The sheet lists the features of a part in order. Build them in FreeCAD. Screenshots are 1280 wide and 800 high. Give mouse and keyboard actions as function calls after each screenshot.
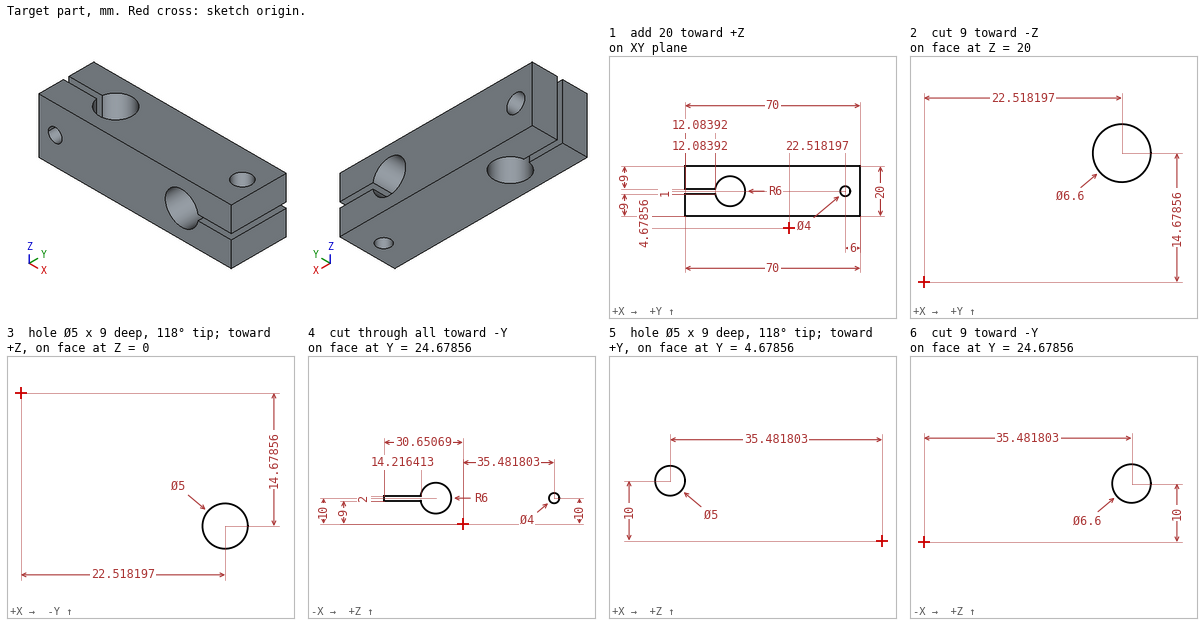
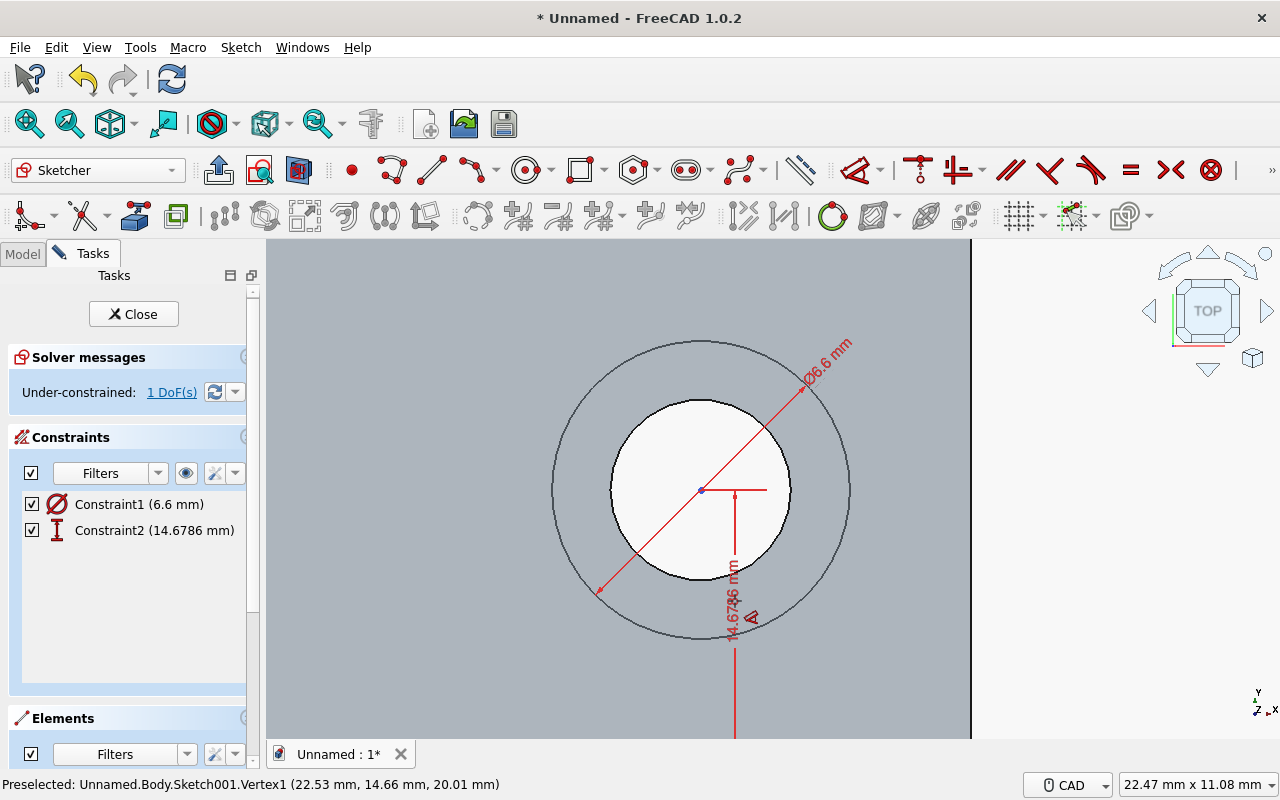
click(701, 490)
click(497, 456)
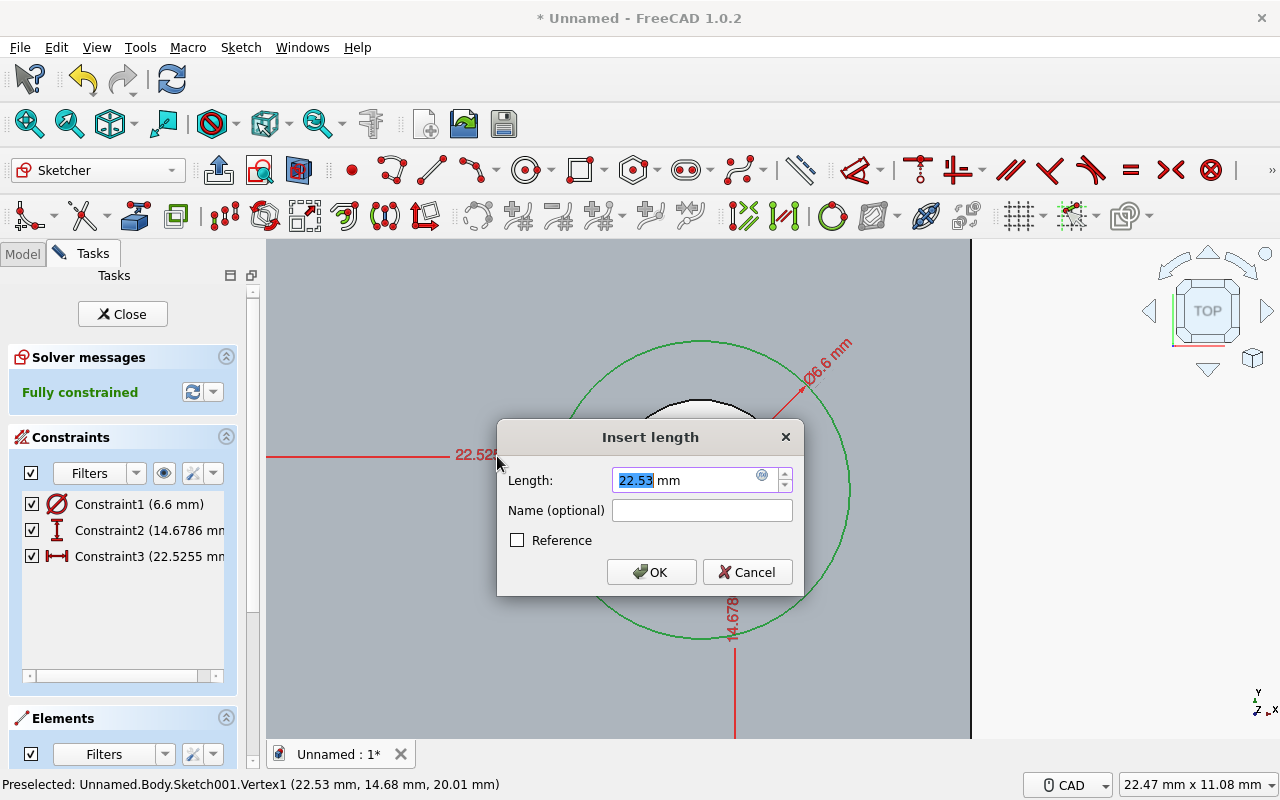
text(22.518197)
key(Return)
key(Escape)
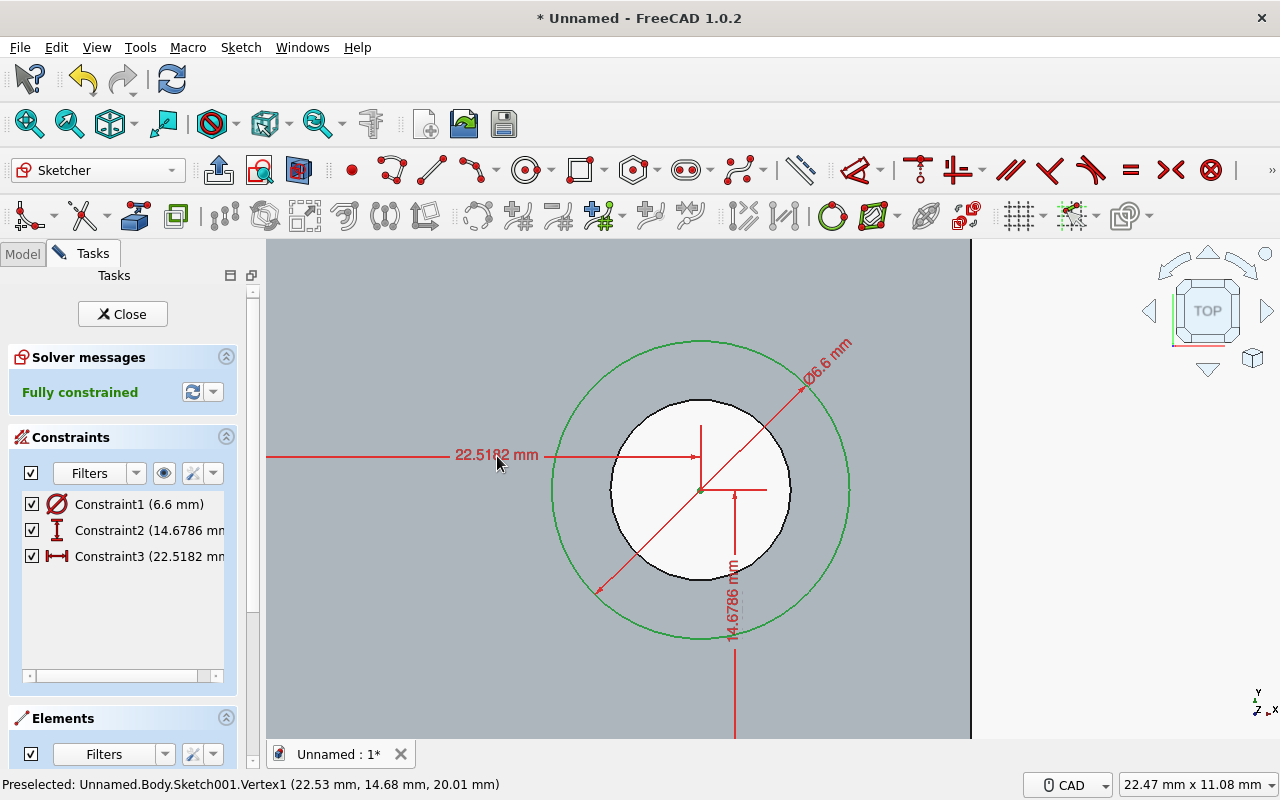
click(123, 314)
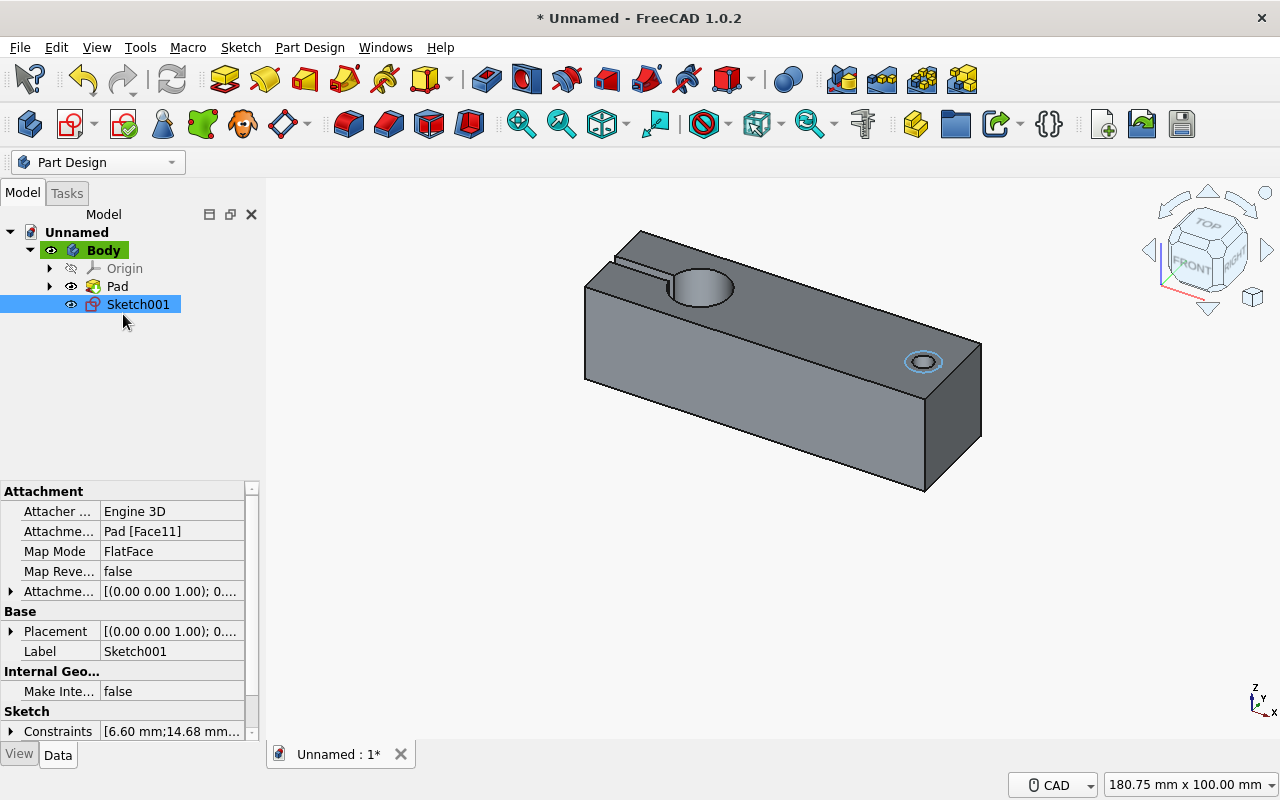
click(488, 80)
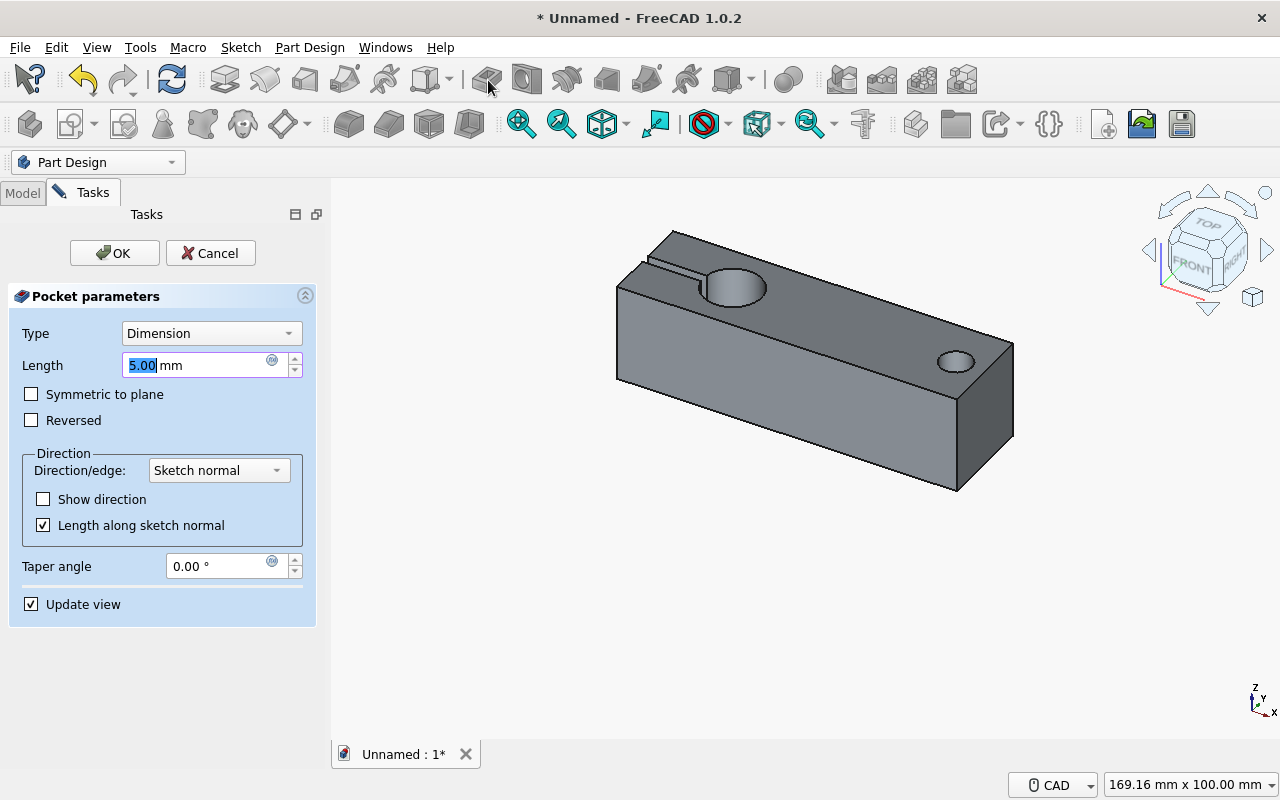
text(9)
key(Tab)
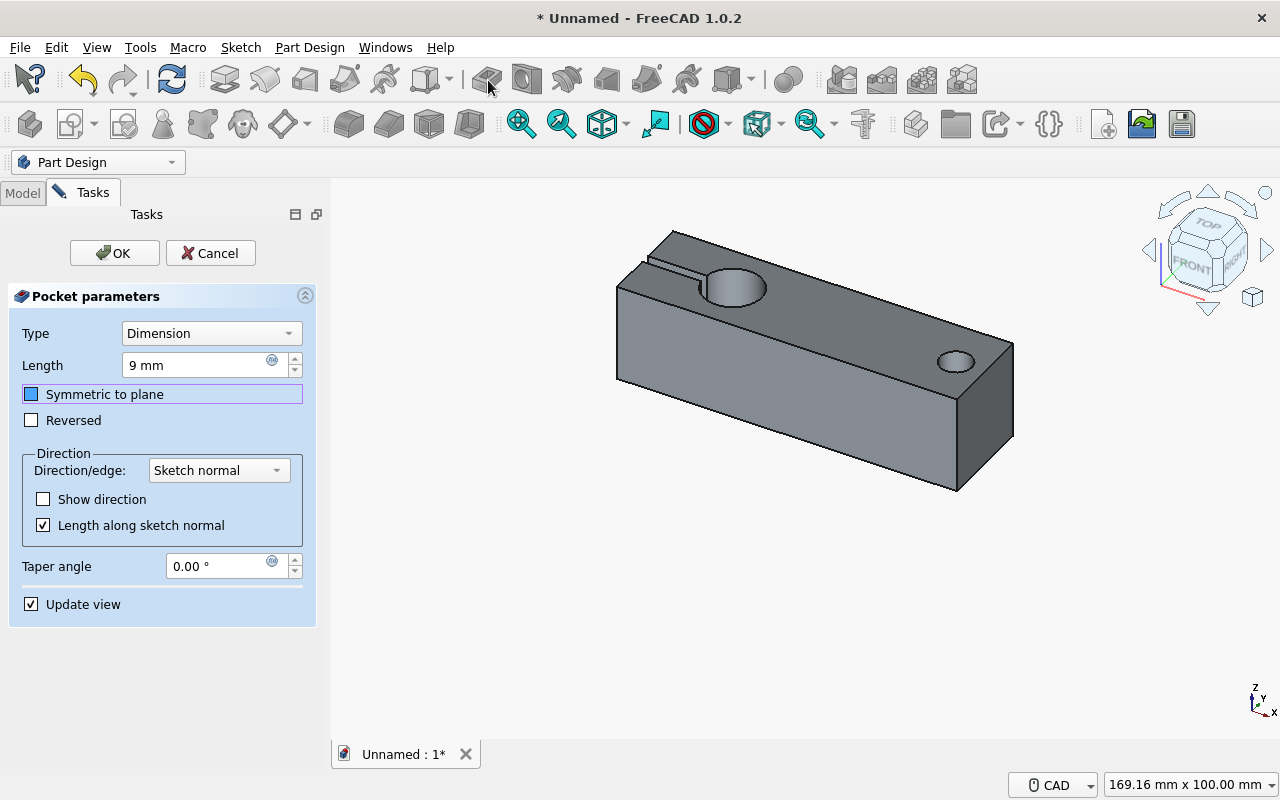
click(115, 253)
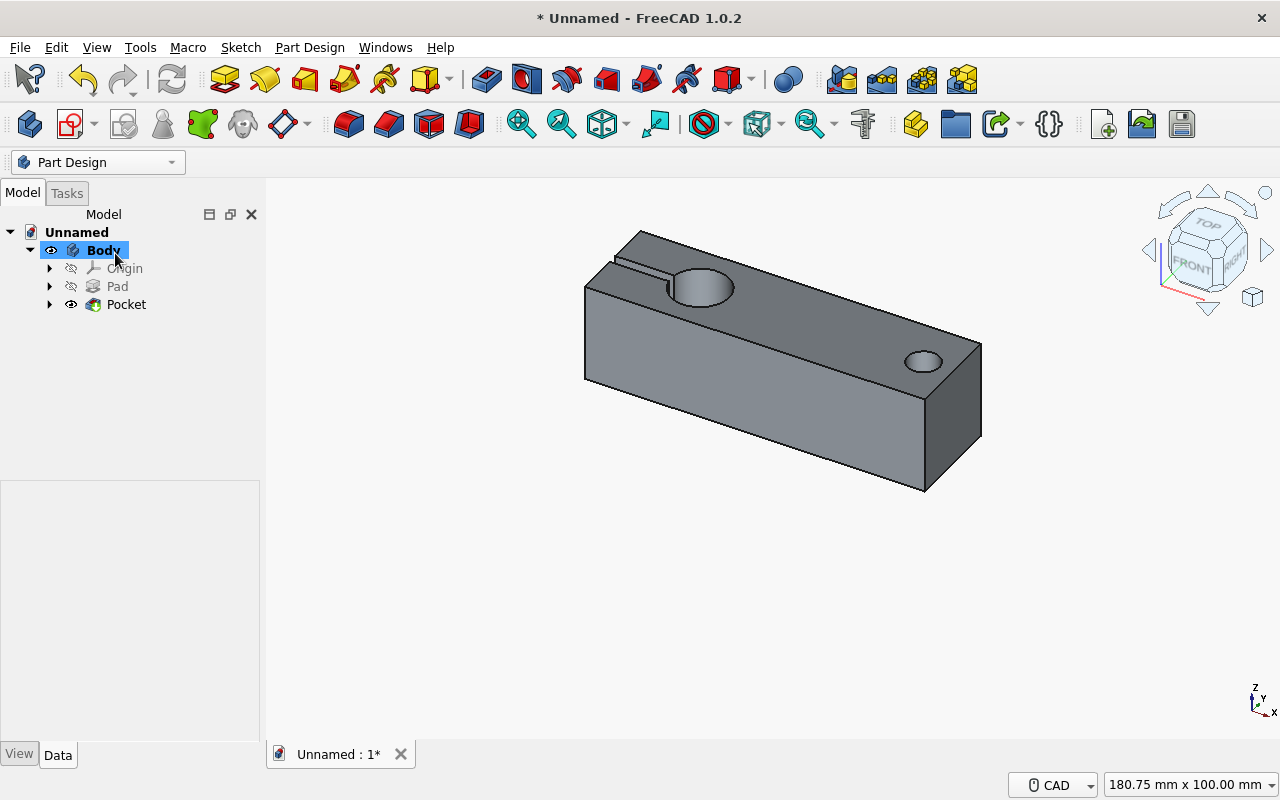
key(5)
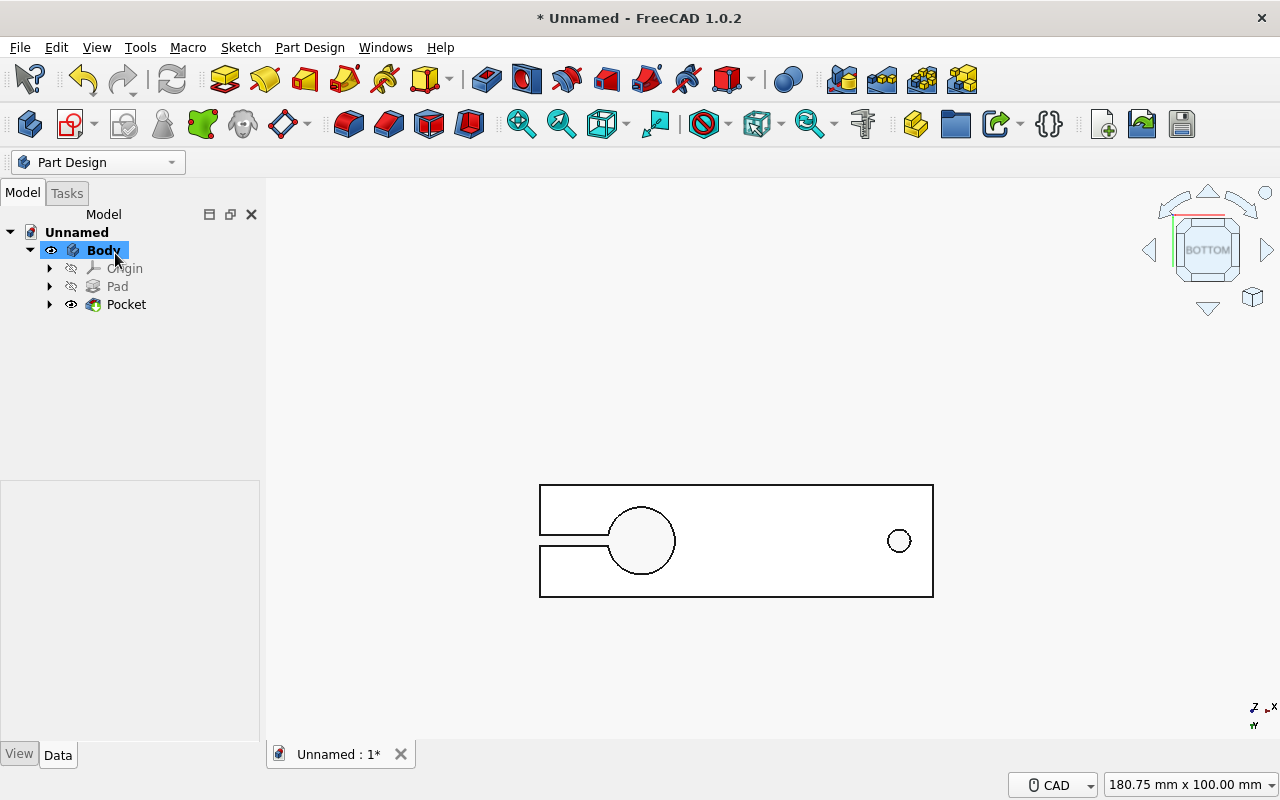
click(522, 124)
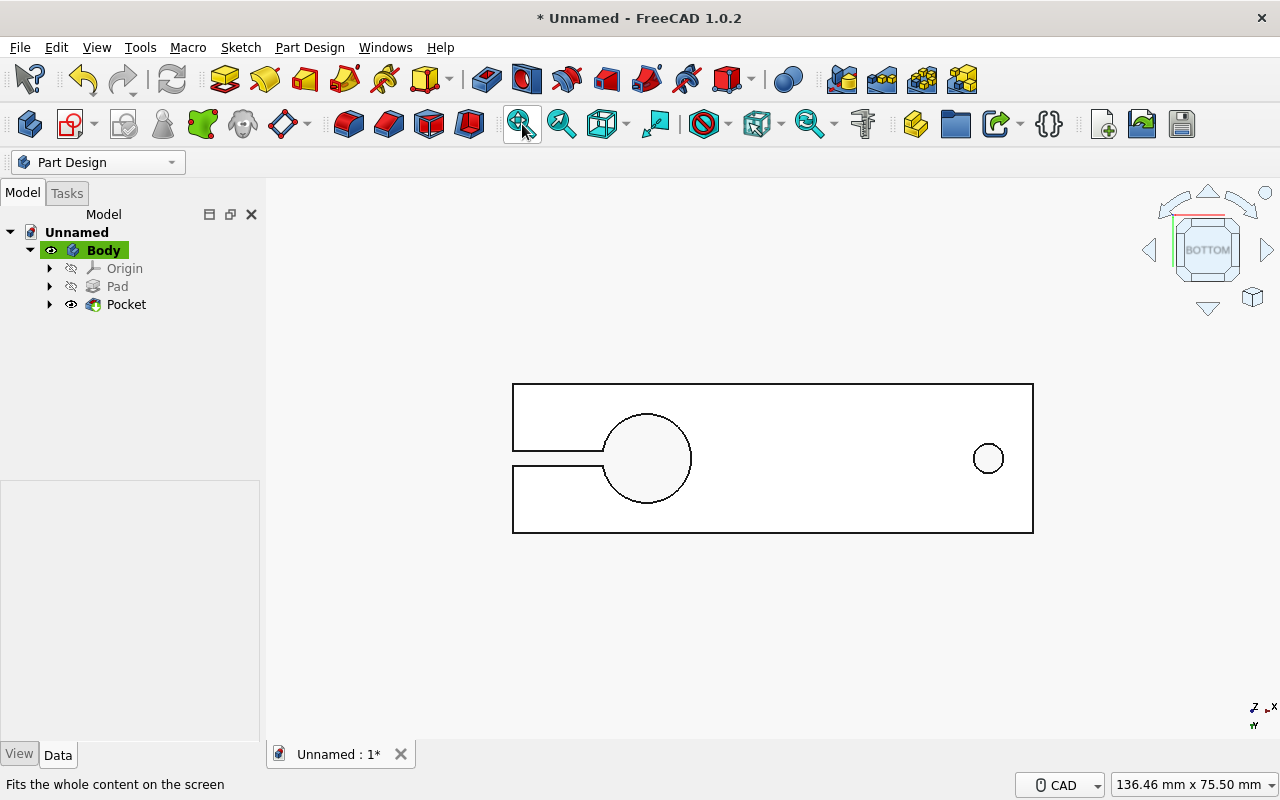
click(847, 457)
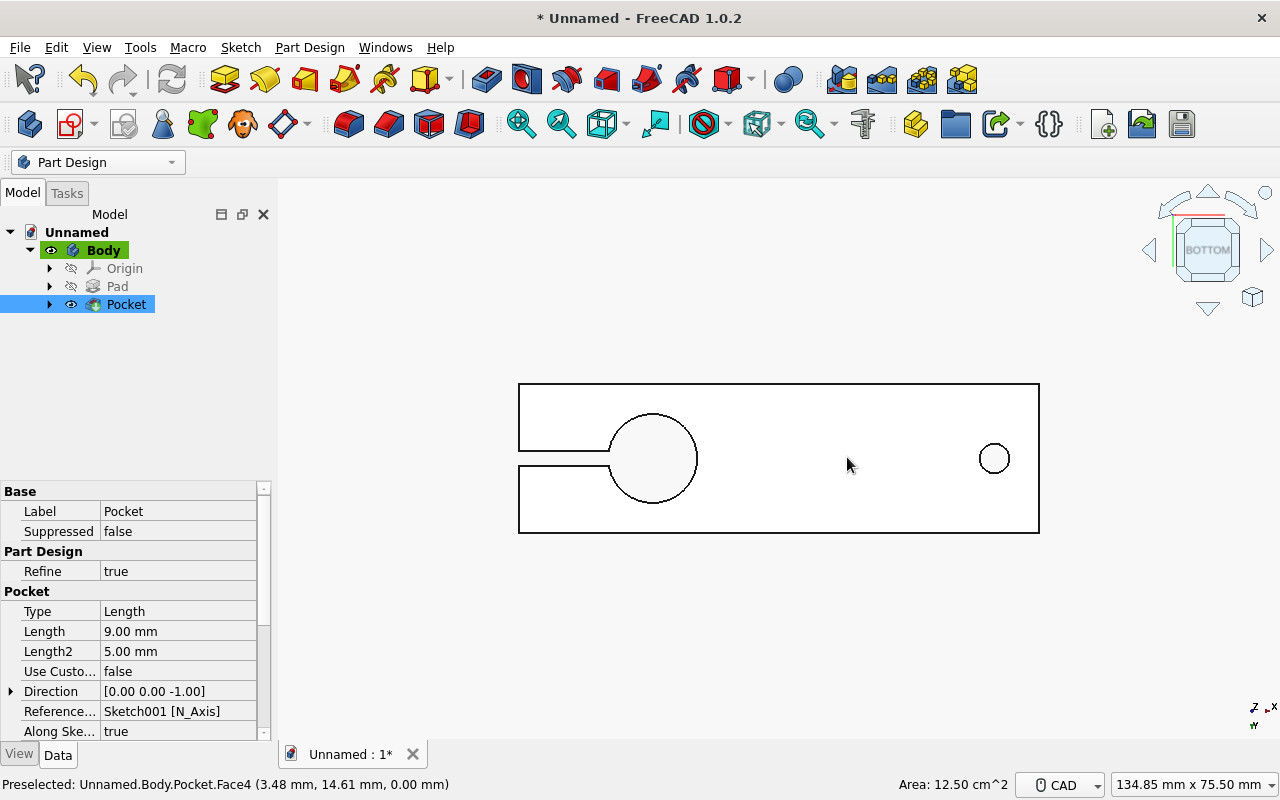
click(70, 124)